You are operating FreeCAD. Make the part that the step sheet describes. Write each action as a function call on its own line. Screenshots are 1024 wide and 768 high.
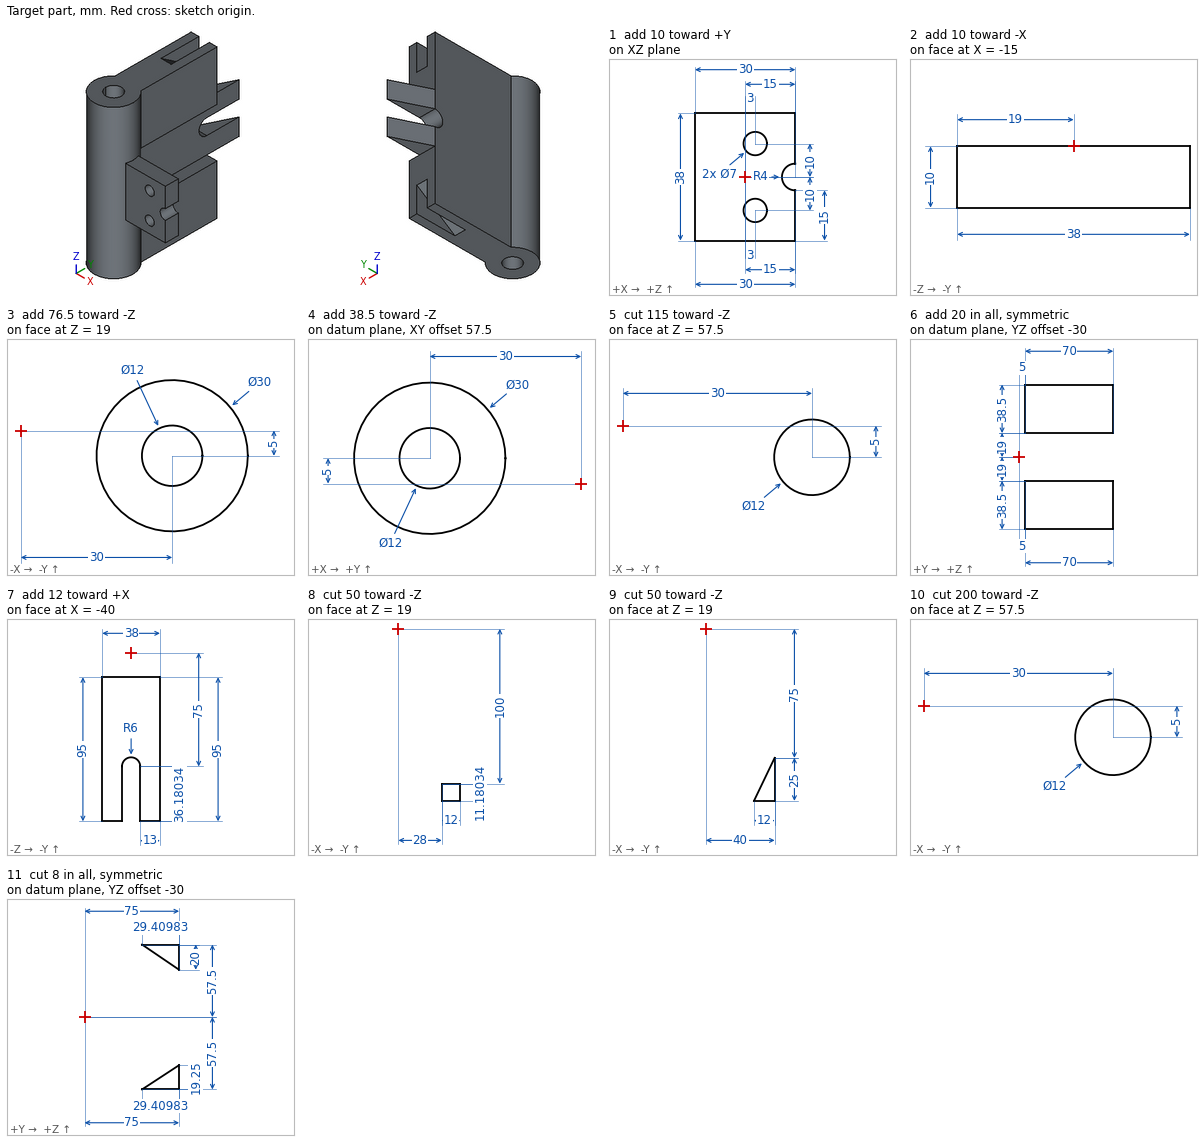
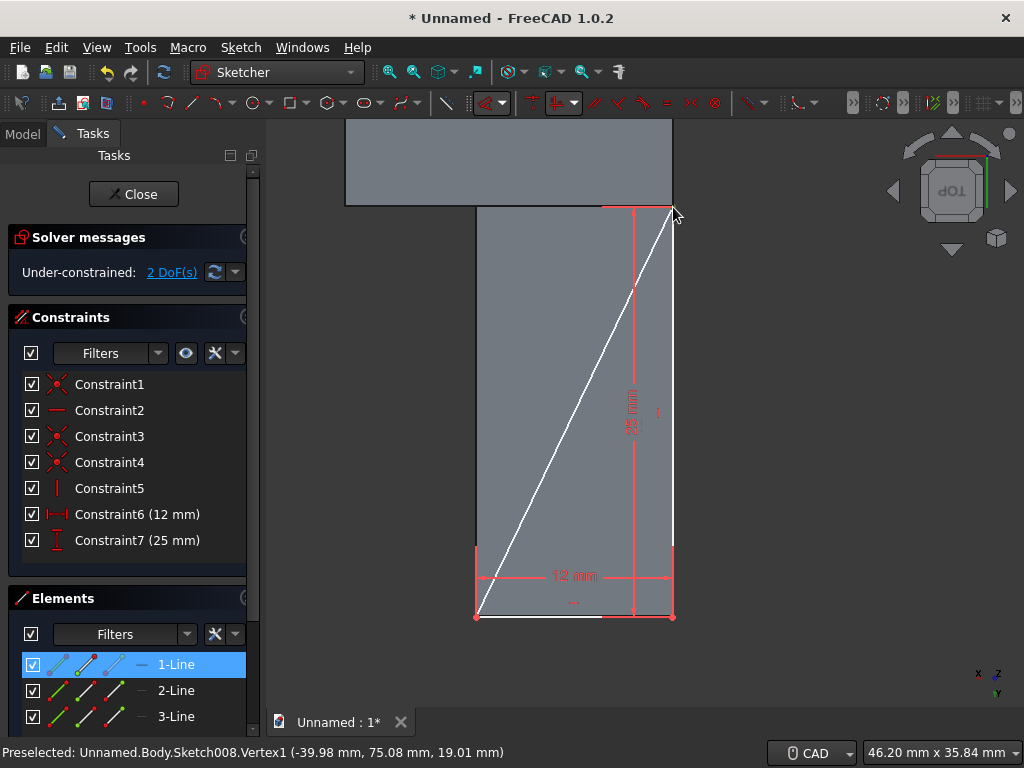
click(504, 104)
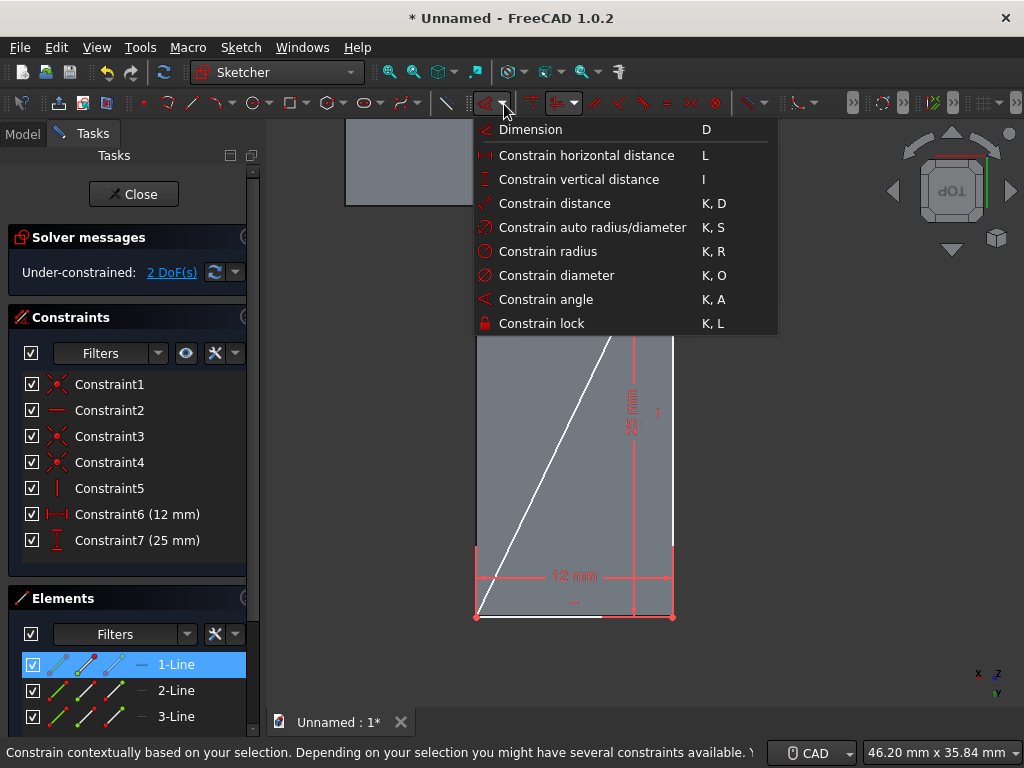
click(626, 155)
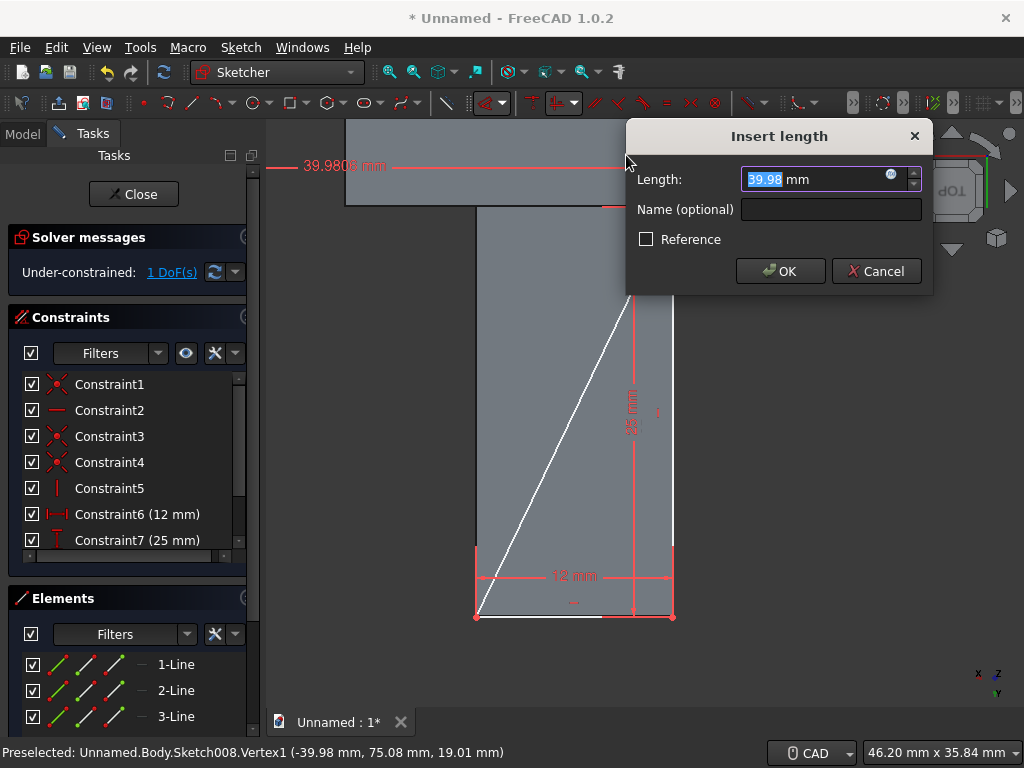
text(40)
key(Return)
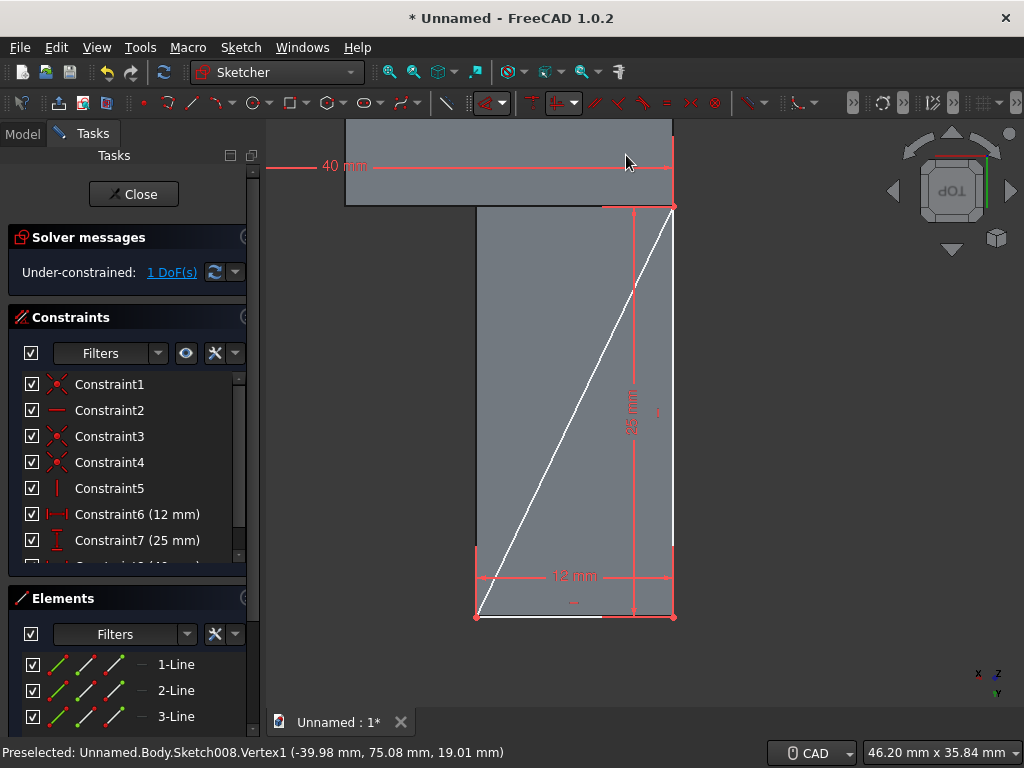
click(673, 207)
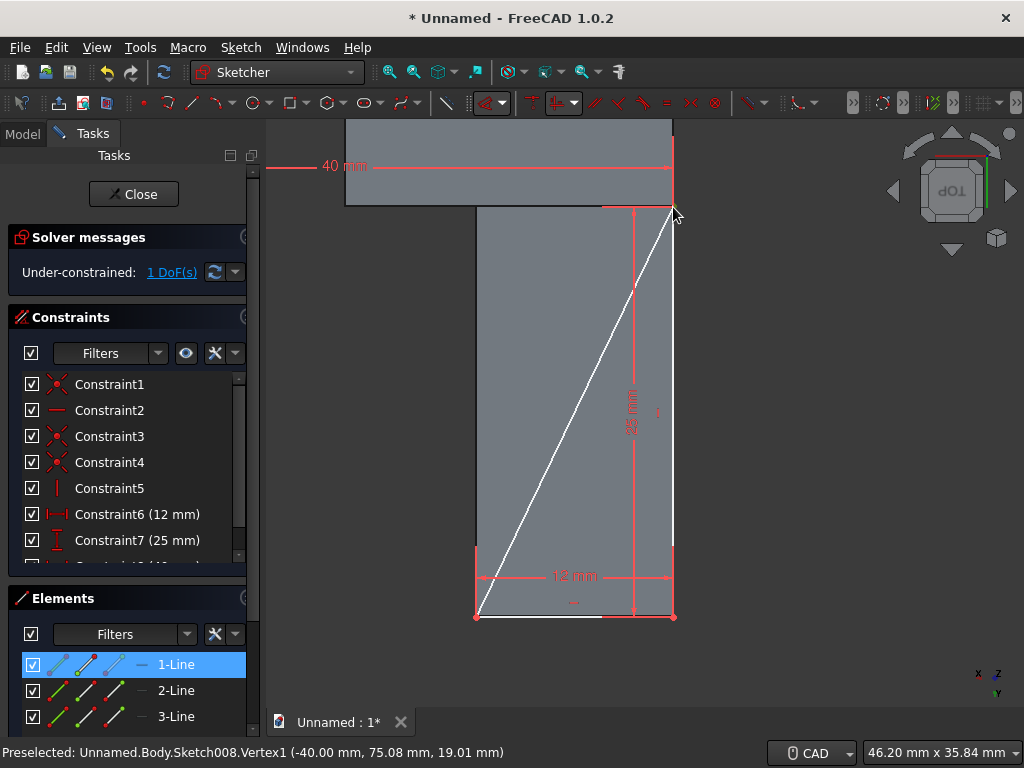
click(504, 104)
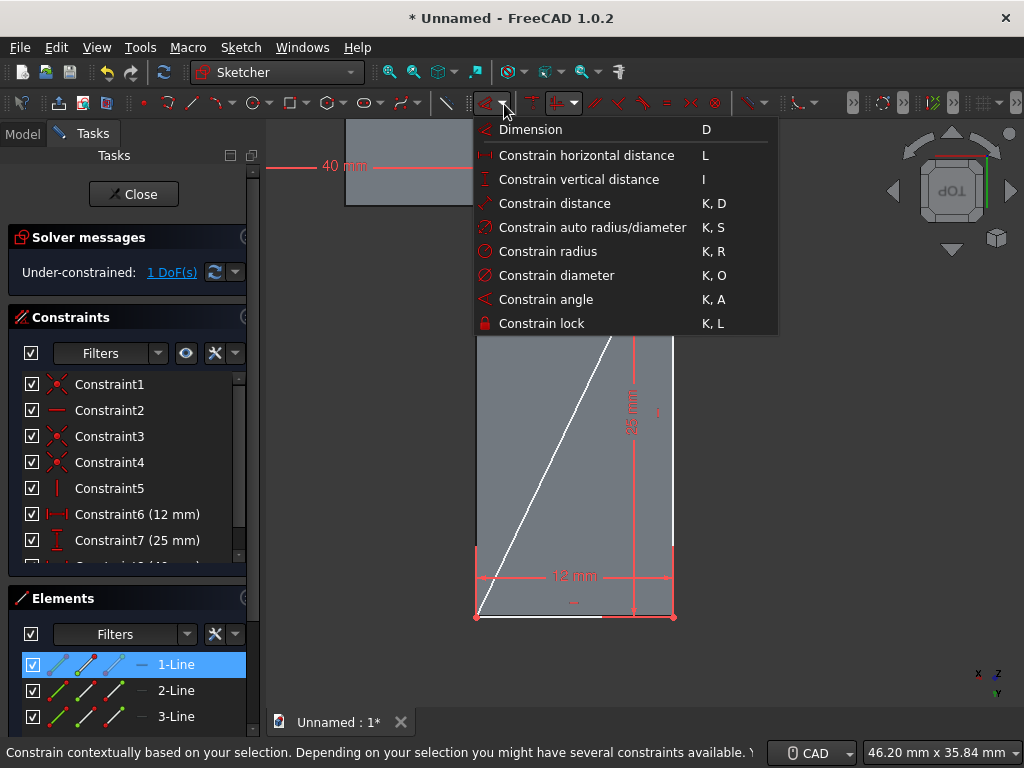
click(626, 179)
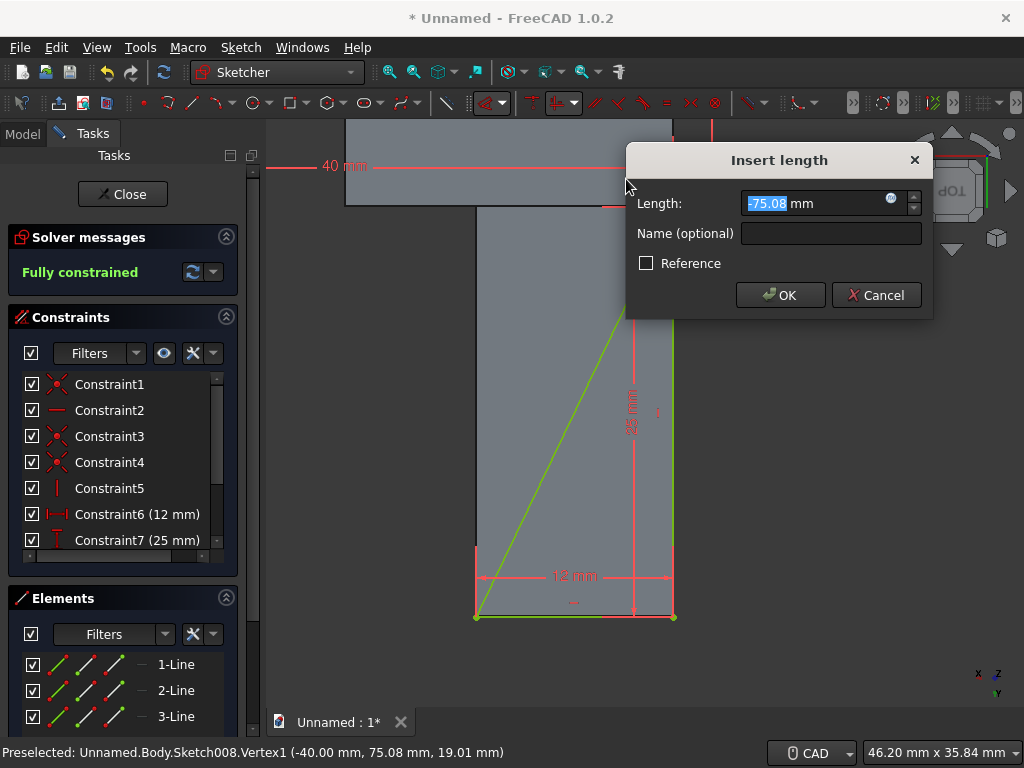
text(-75)
key(Return)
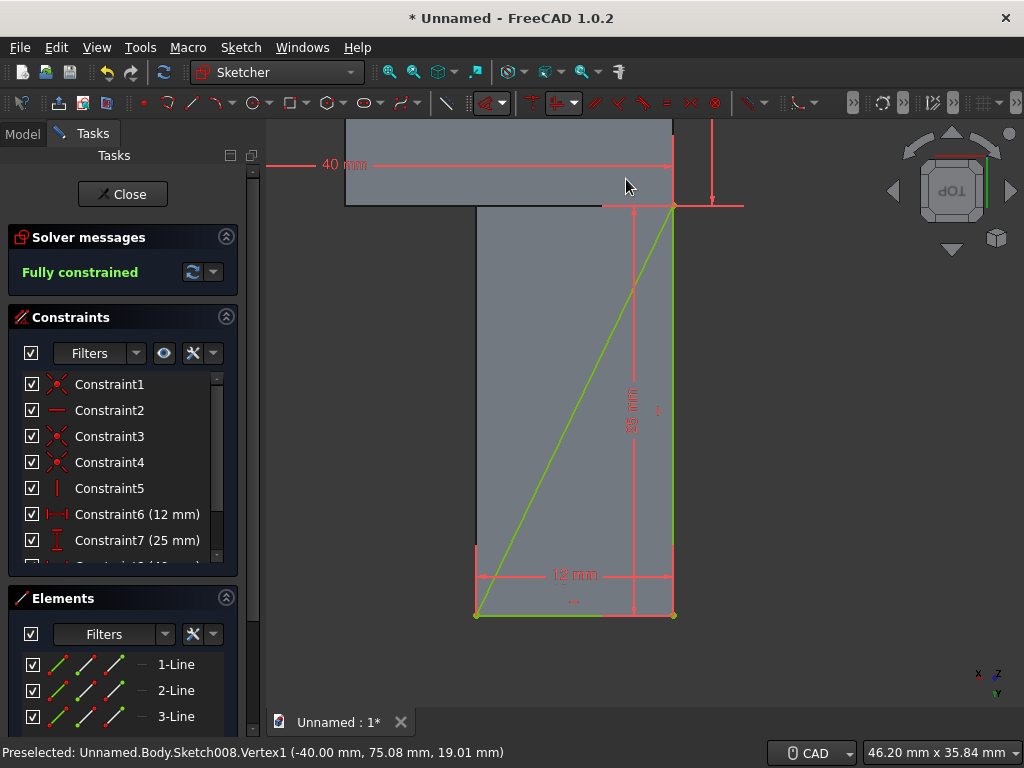
click(123, 194)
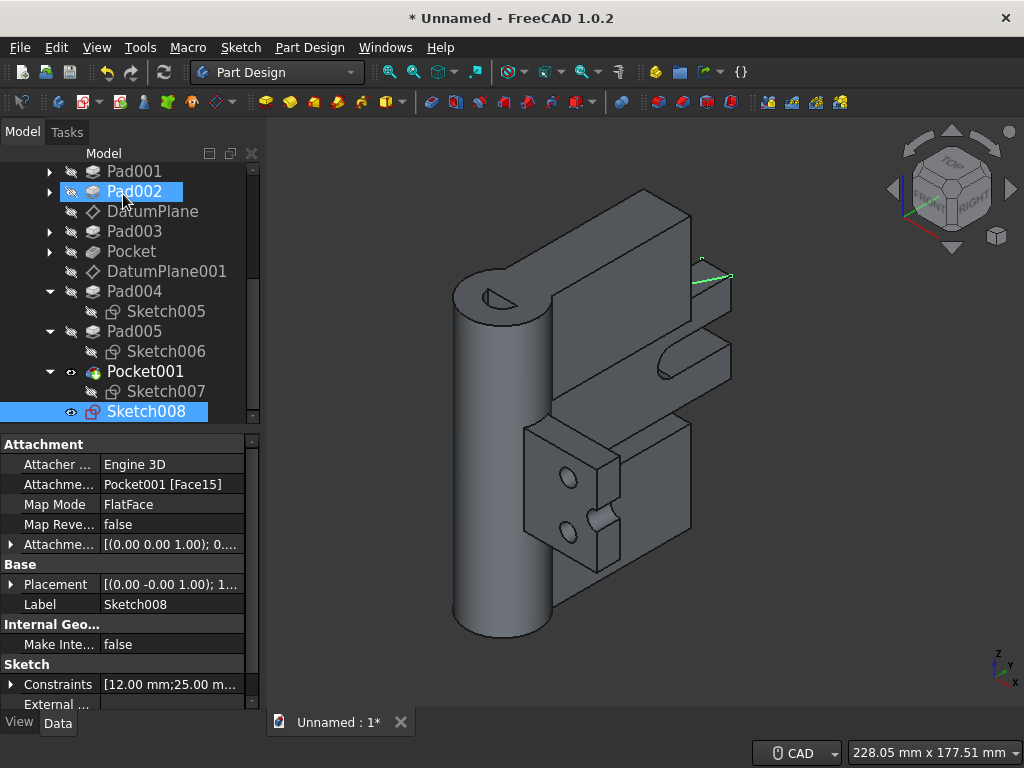
click(432, 102)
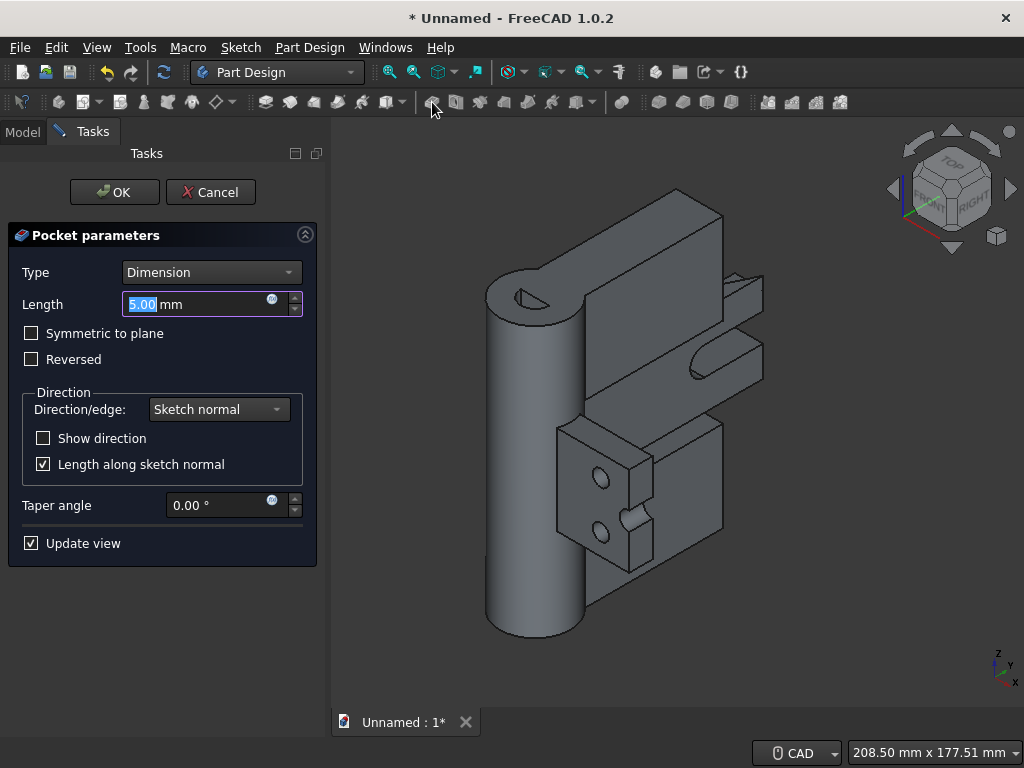
text(50)
key(Tab)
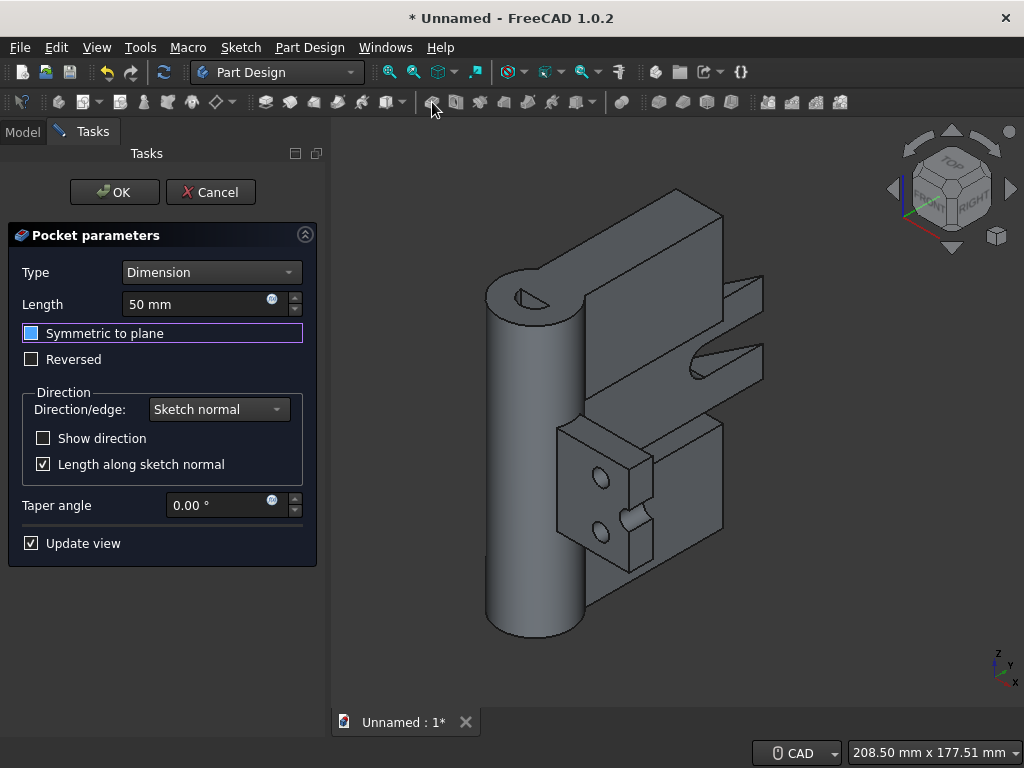
click(115, 192)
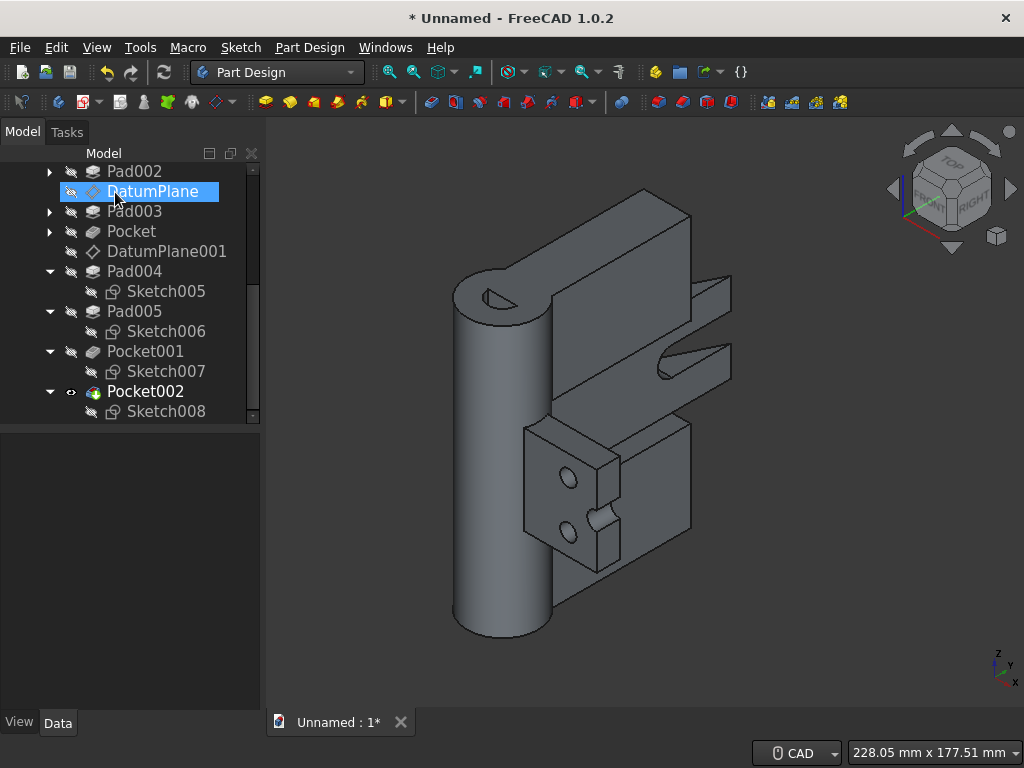
click(624, 226)